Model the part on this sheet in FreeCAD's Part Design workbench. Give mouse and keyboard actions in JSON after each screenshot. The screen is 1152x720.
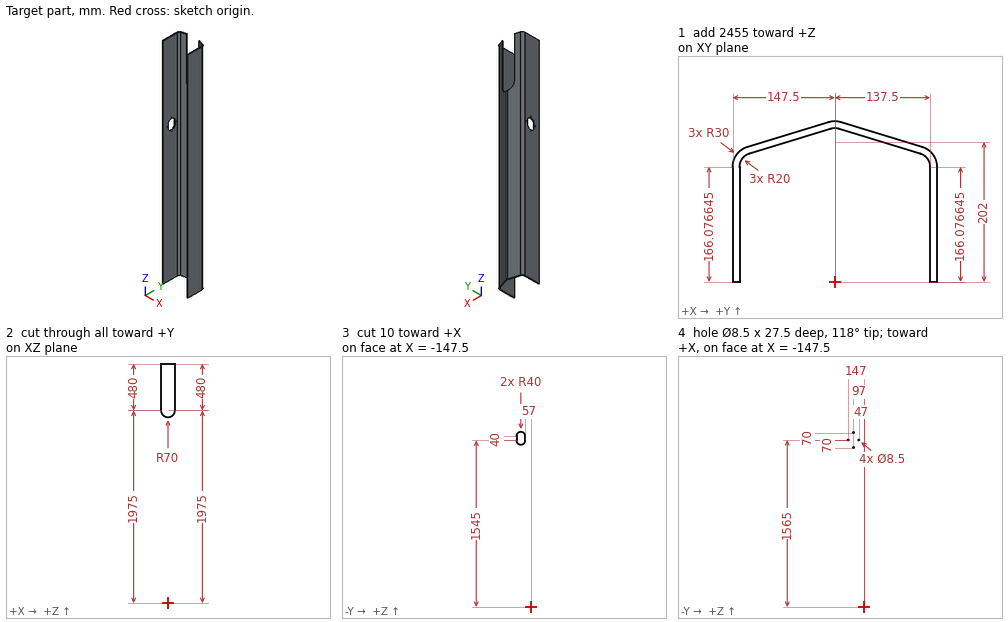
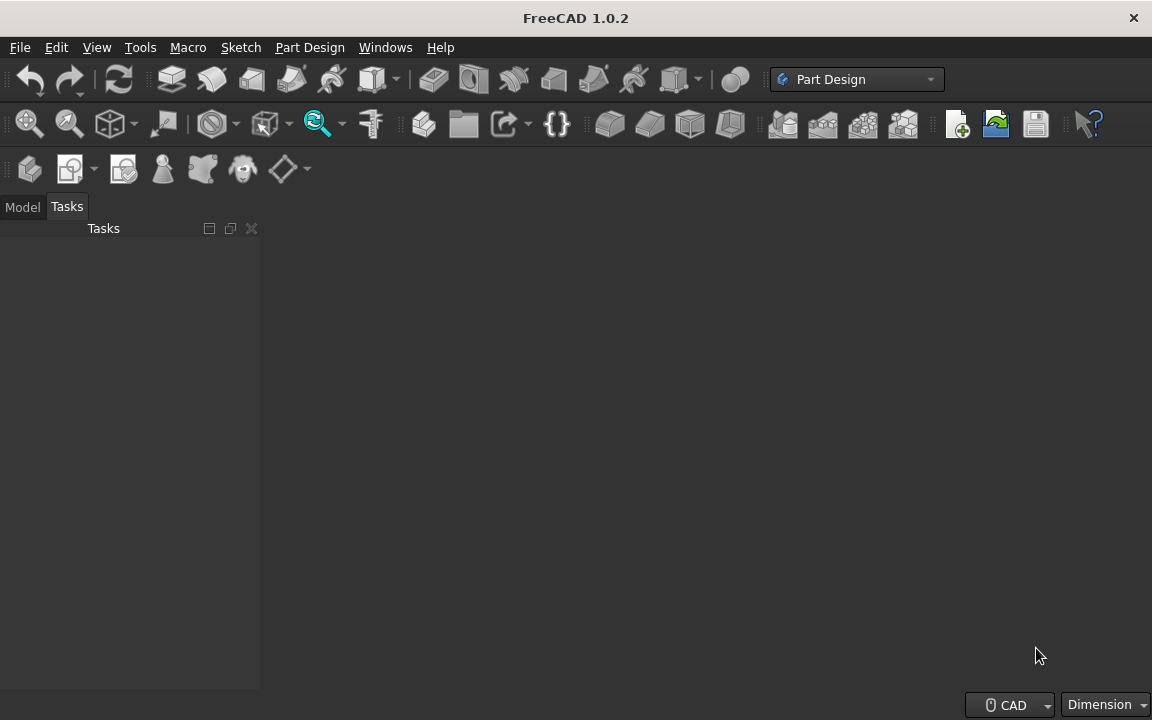
{"action": "left_click", "coordinate": [956, 124]}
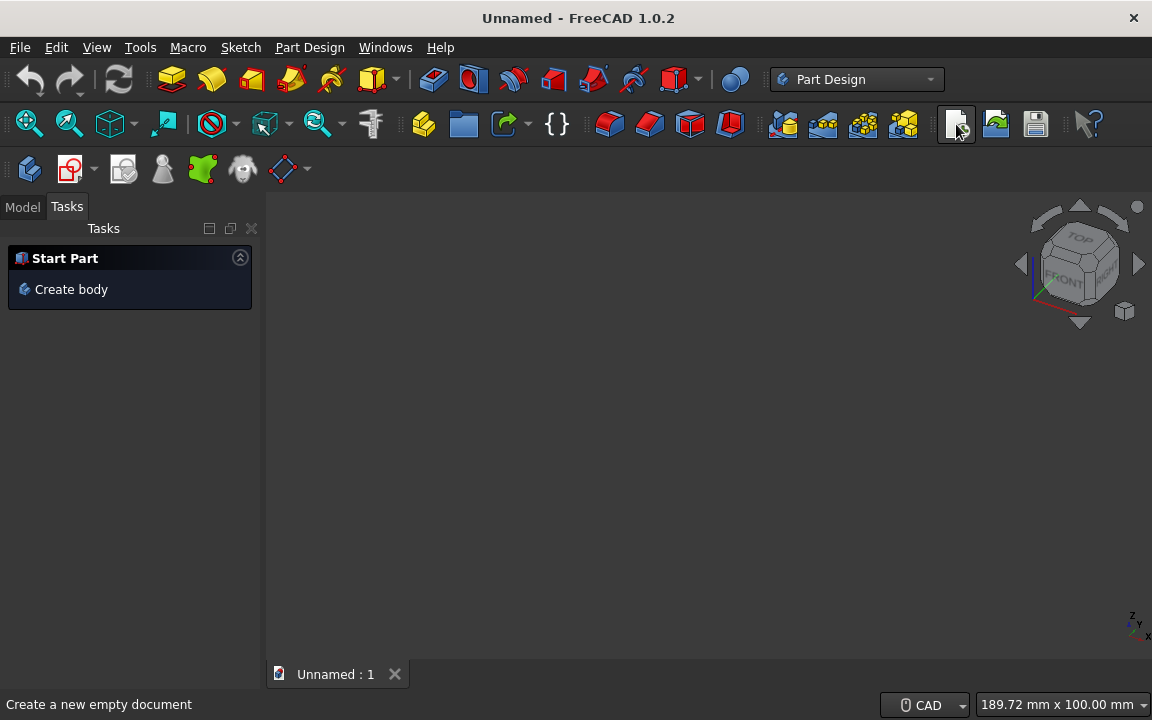
{"action": "left_click", "coordinate": [70, 170]}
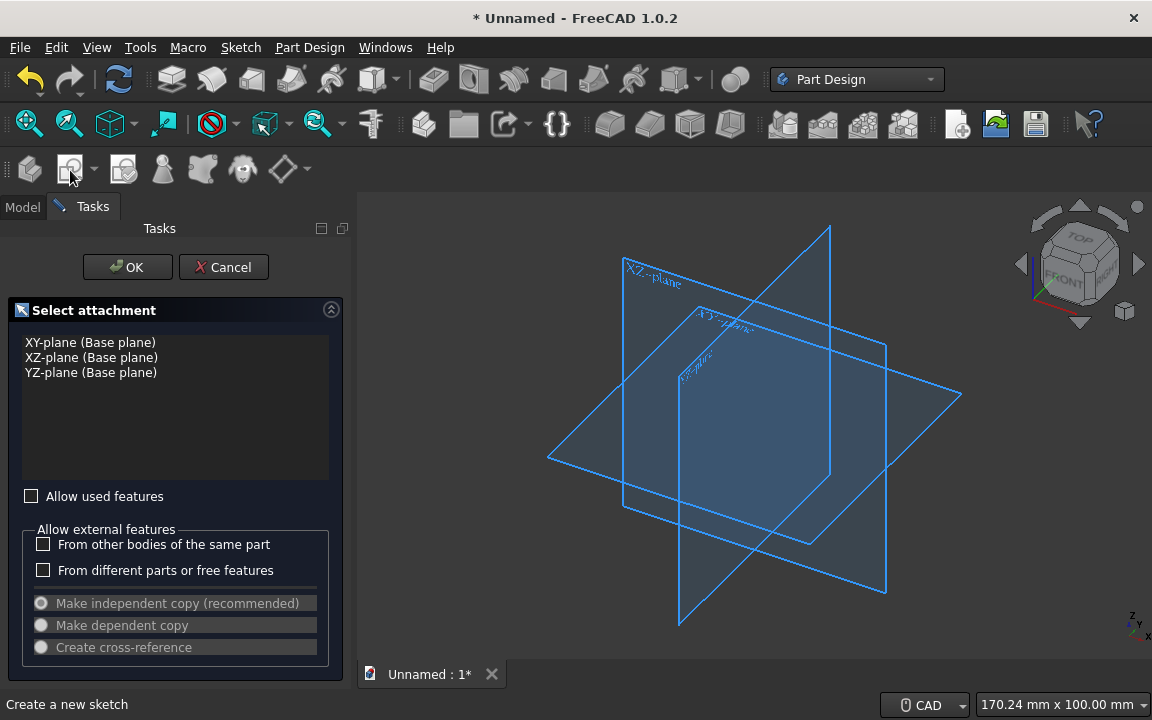
{"action": "left_click", "coordinate": [82, 342]}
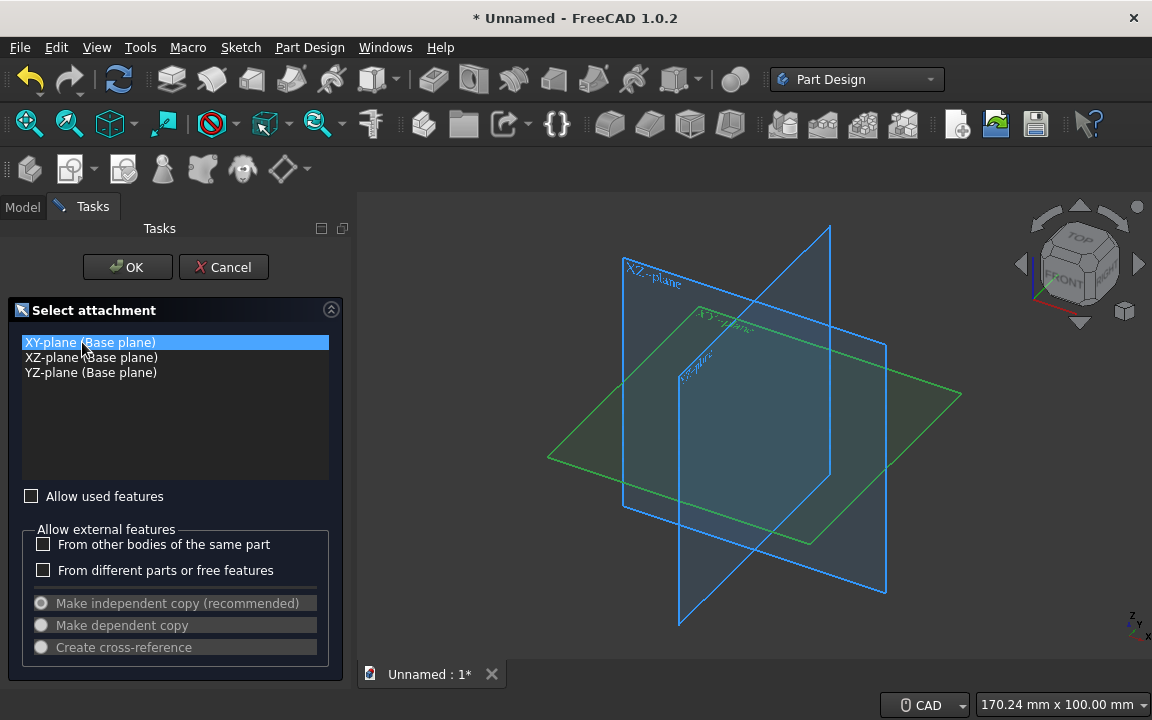
{"action": "left_click", "coordinate": [128, 267]}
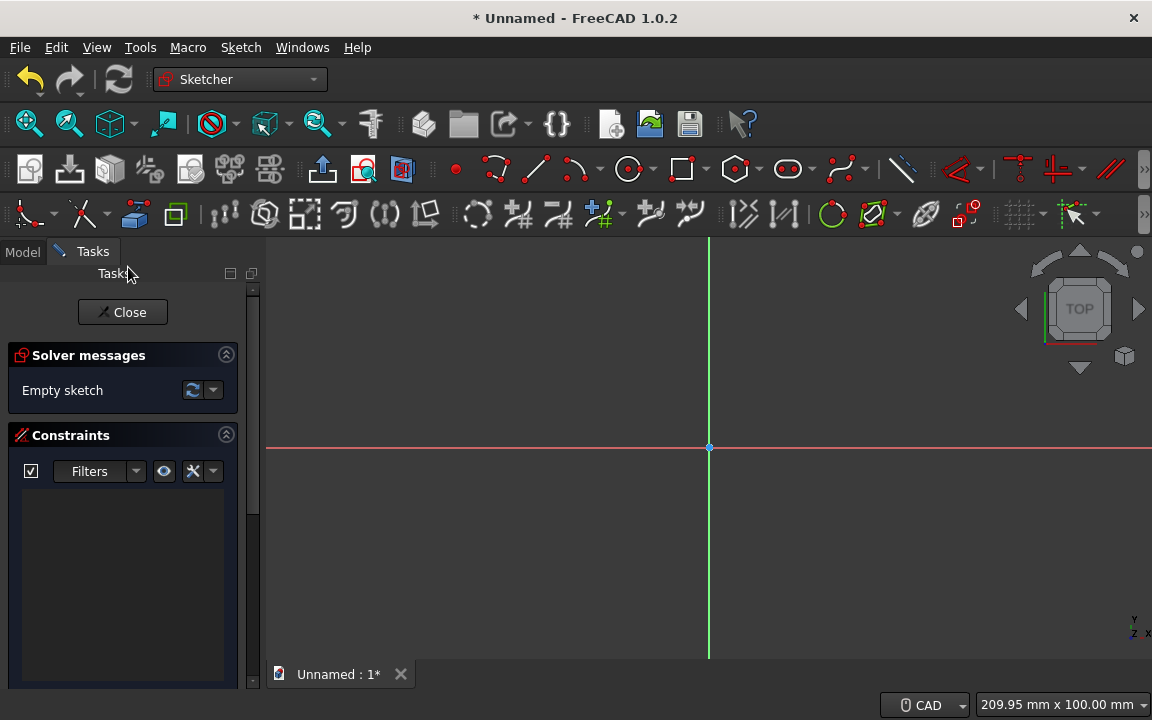
{"action": "scroll", "coordinate": [618, 608], "scroll_direction": "down", "scroll_amount": 7}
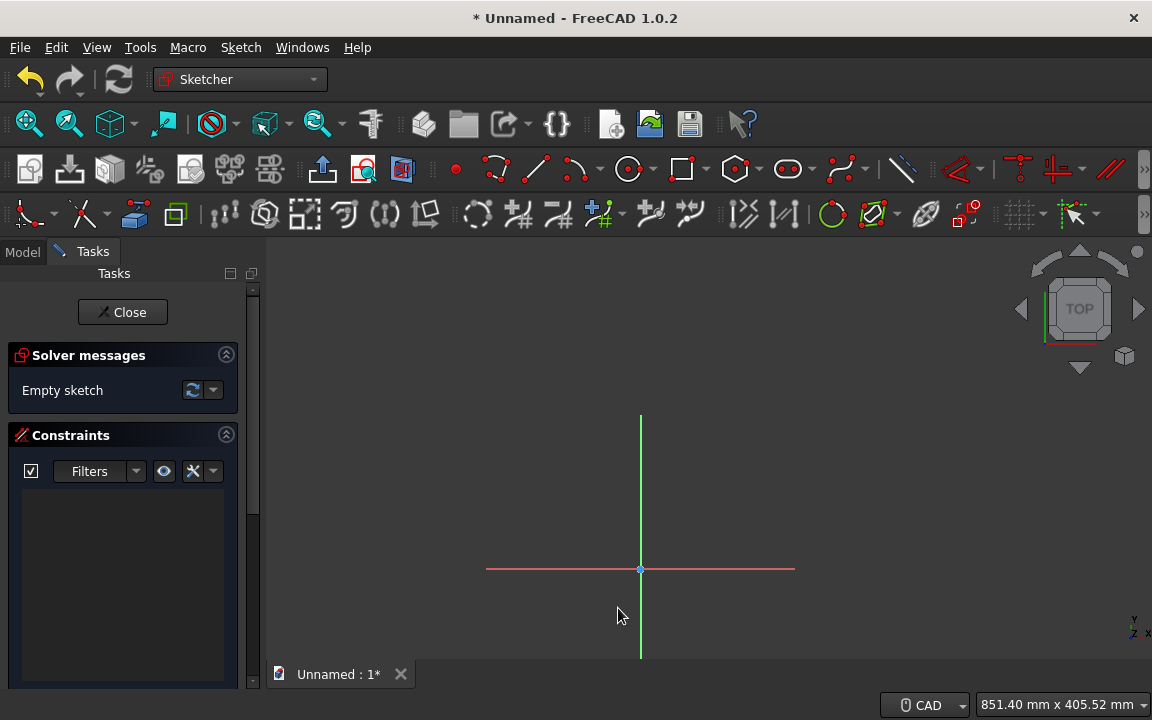
{"action": "left_click", "coordinate": [496, 170]}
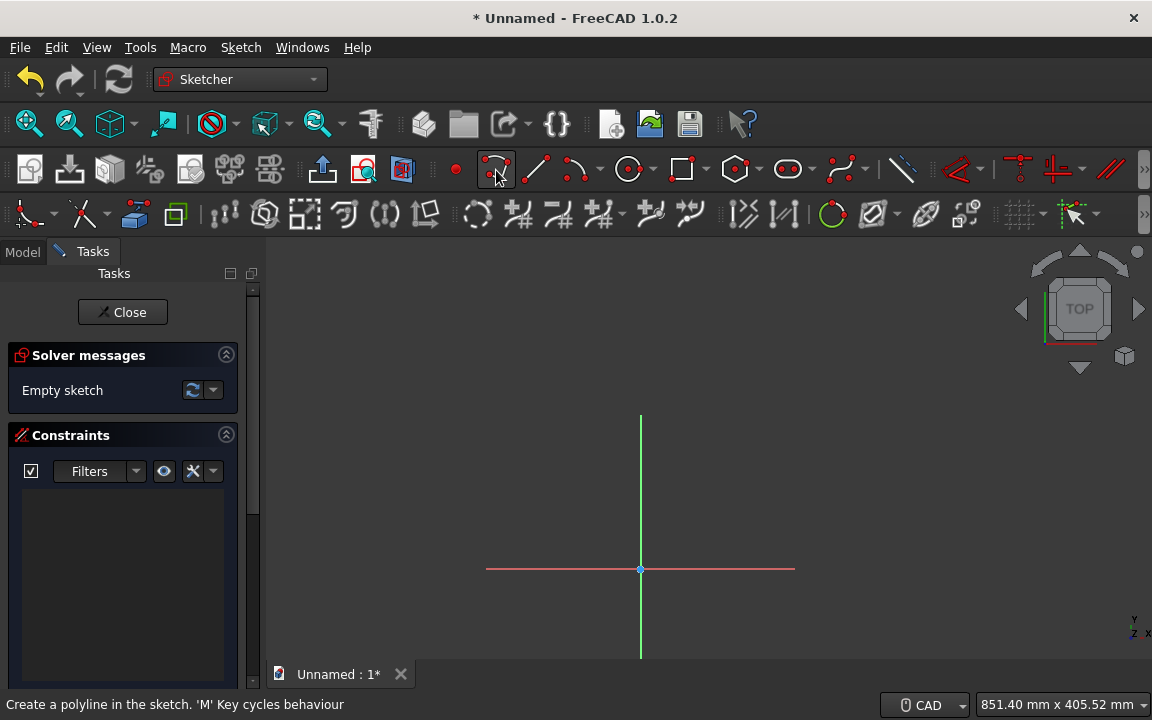
{"action": "left_click", "coordinate": [487, 396]}
{"action": "left_click", "coordinate": [487, 569]}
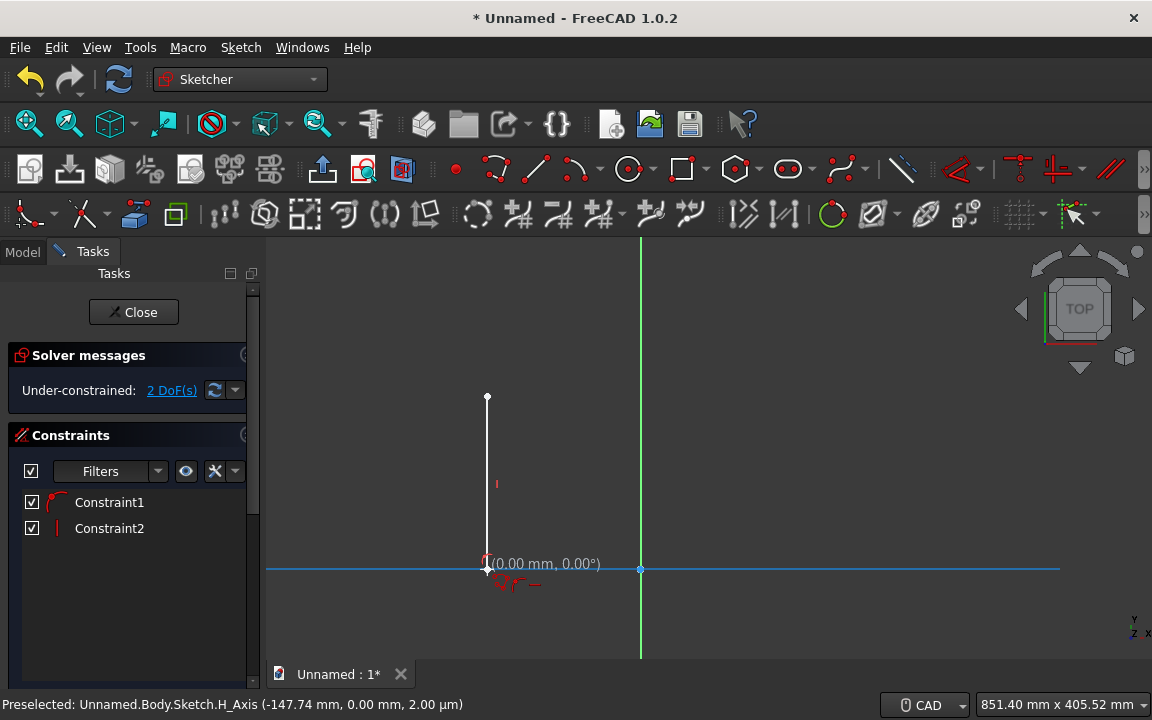
{"action": "scroll", "coordinate": [498, 569], "scroll_direction": "up", "scroll_amount": 3}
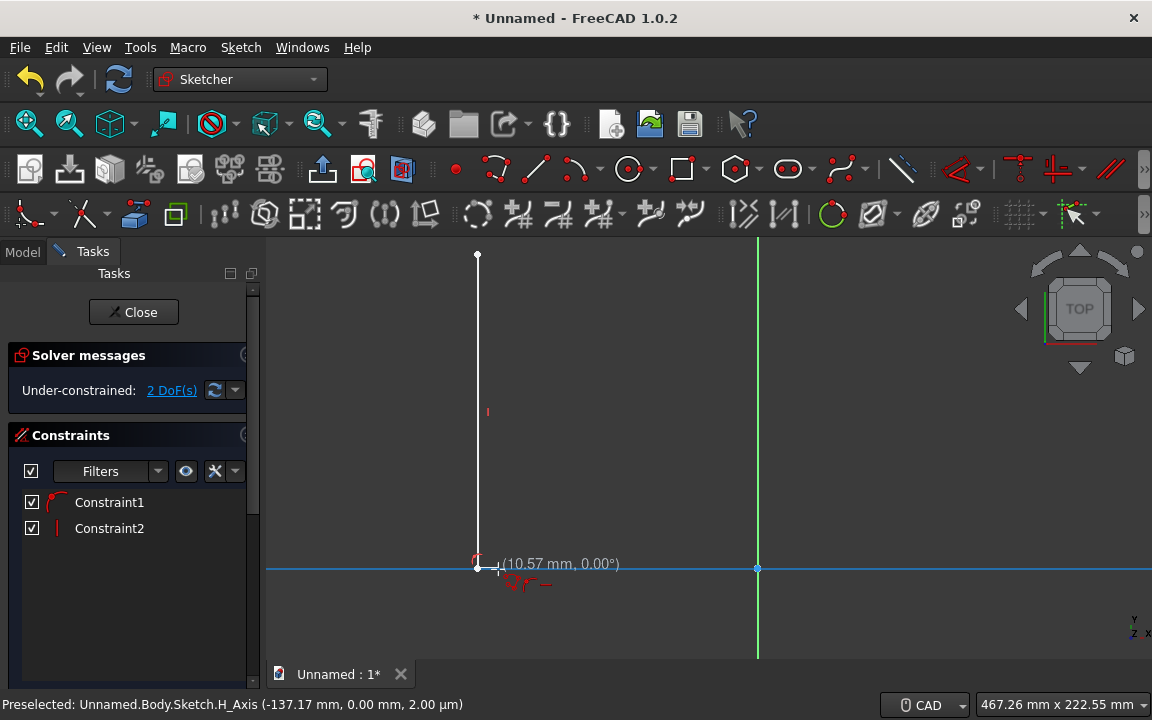
{"action": "left_click", "coordinate": [497, 560]}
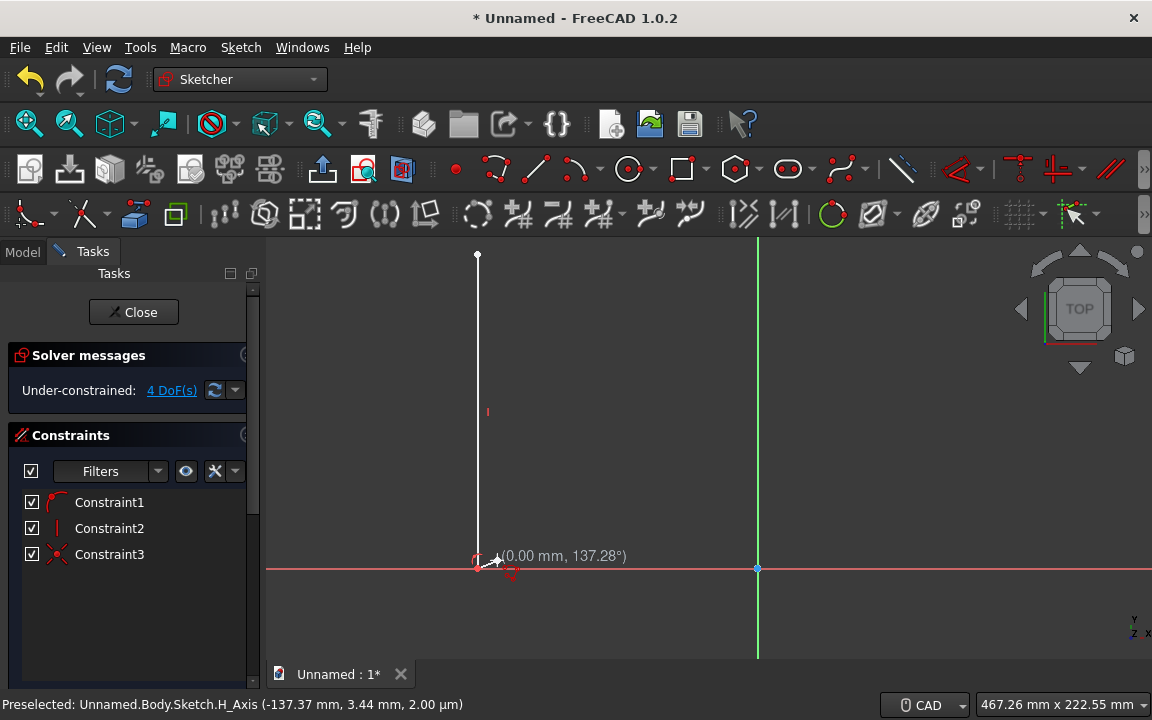
{"action": "scroll", "coordinate": [498, 569], "scroll_direction": "down", "scroll_amount": 3}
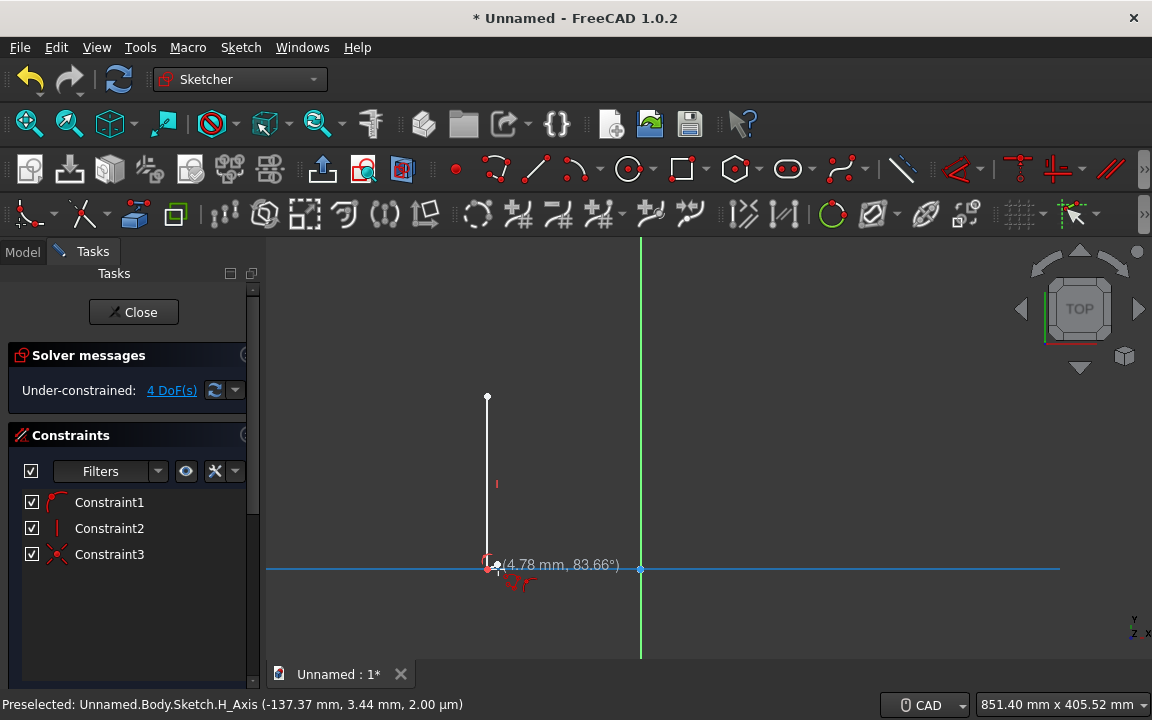
{"action": "scroll", "coordinate": [498, 396], "scroll_direction": "up", "scroll_amount": 3}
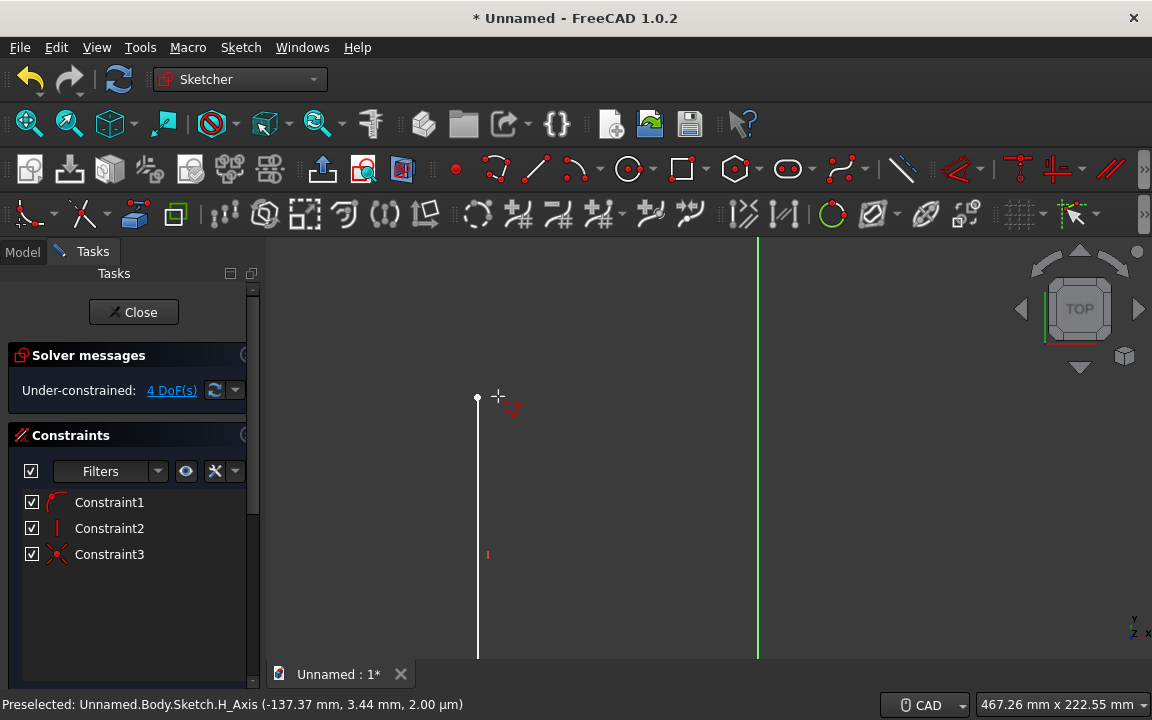
{"action": "left_click", "coordinate": [497, 396]}
{"action": "right_click", "coordinate": [497, 396]}